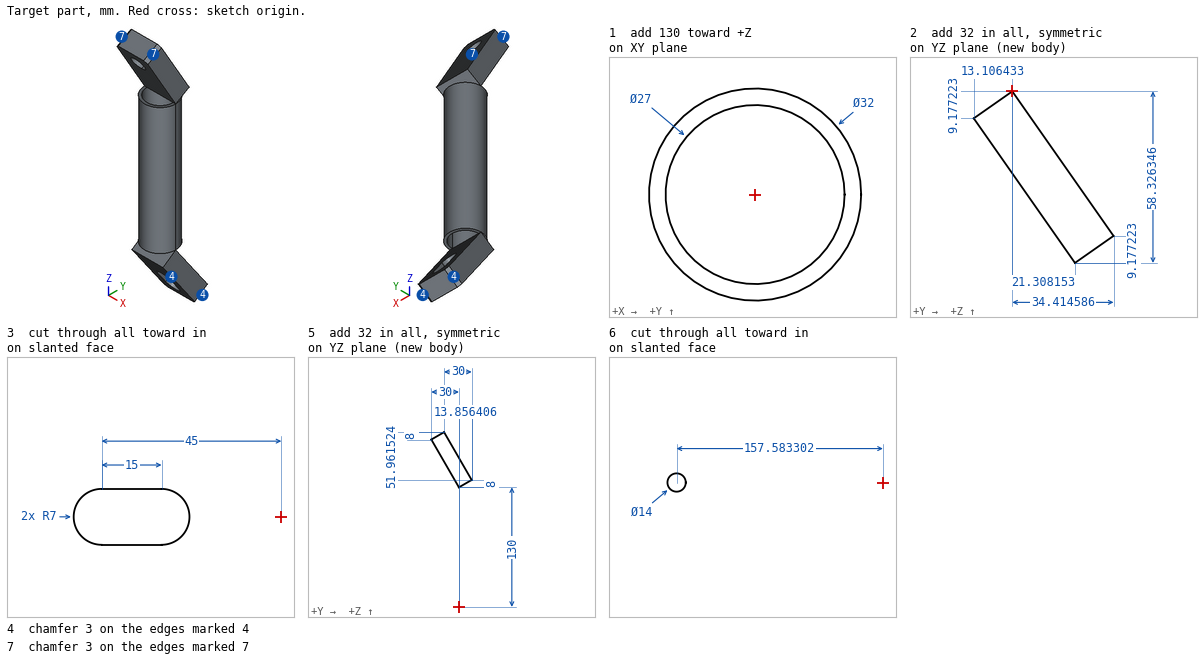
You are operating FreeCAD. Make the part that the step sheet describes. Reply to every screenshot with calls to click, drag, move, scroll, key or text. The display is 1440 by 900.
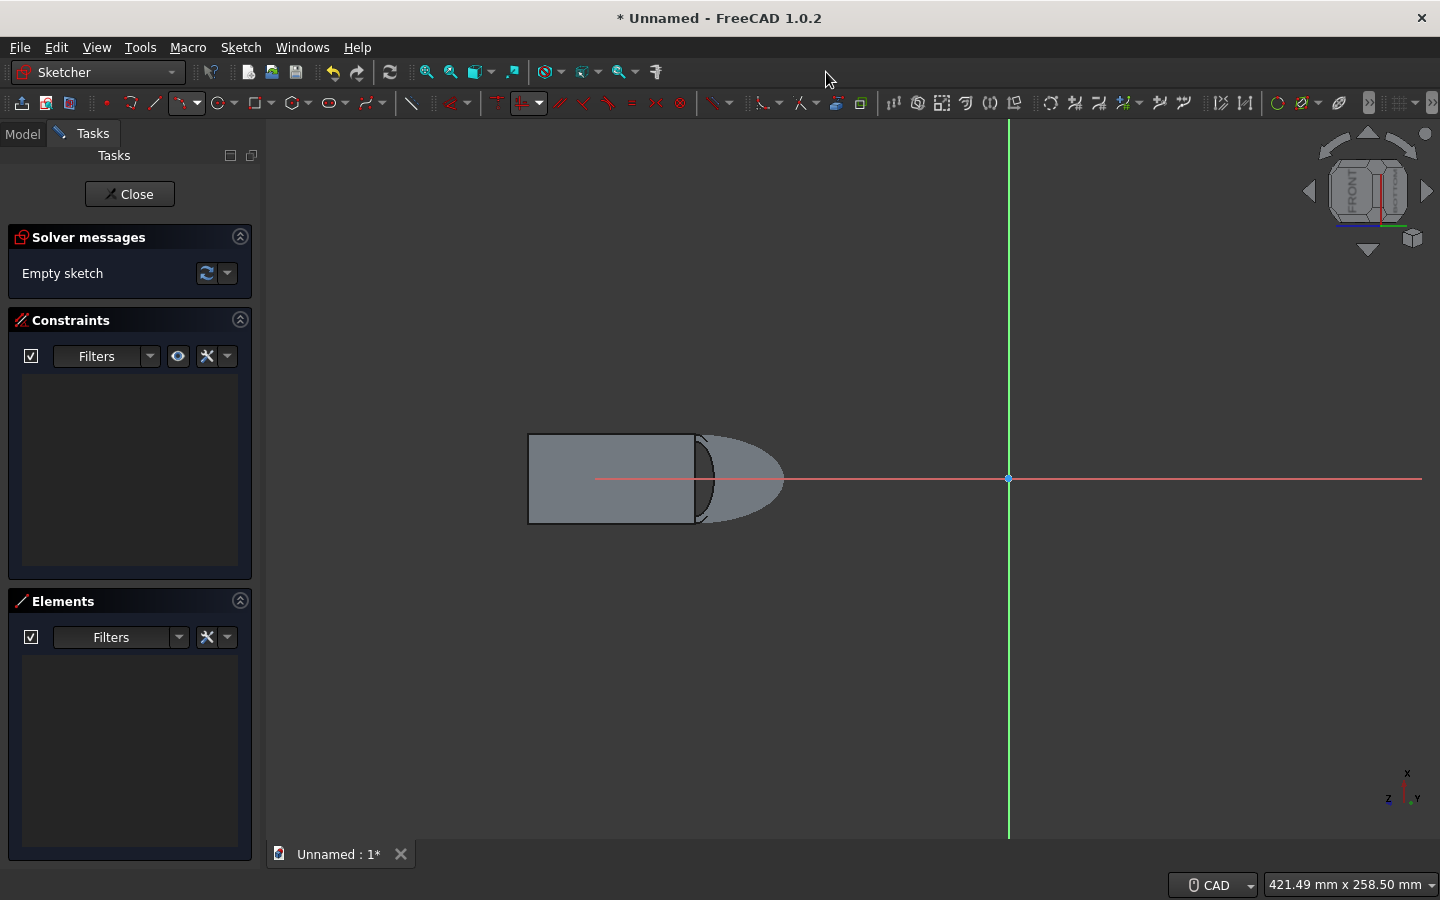
scroll(548, 479, up, 12)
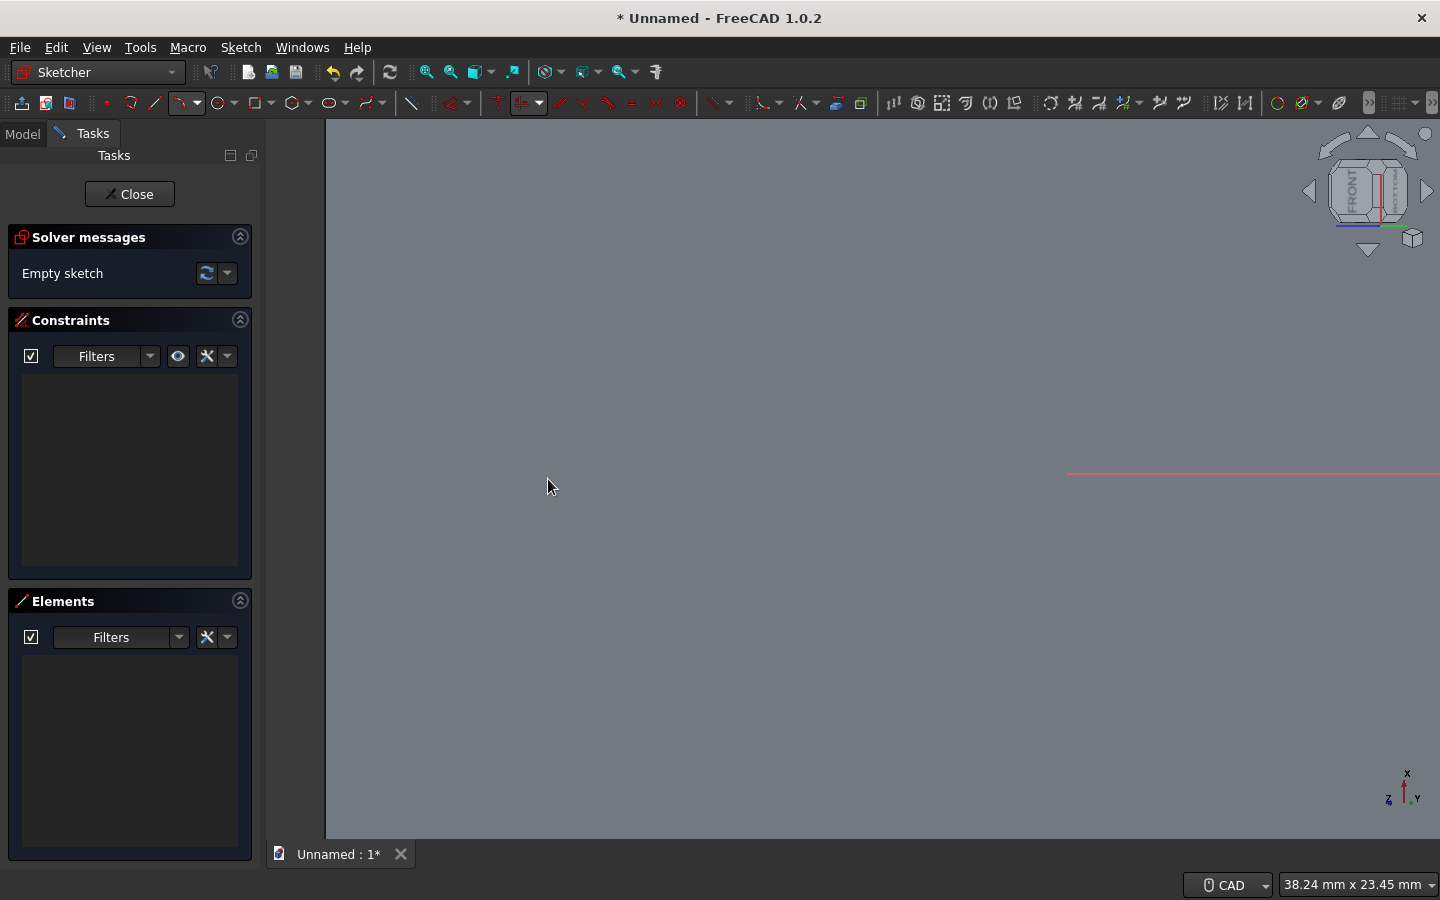
click(218, 104)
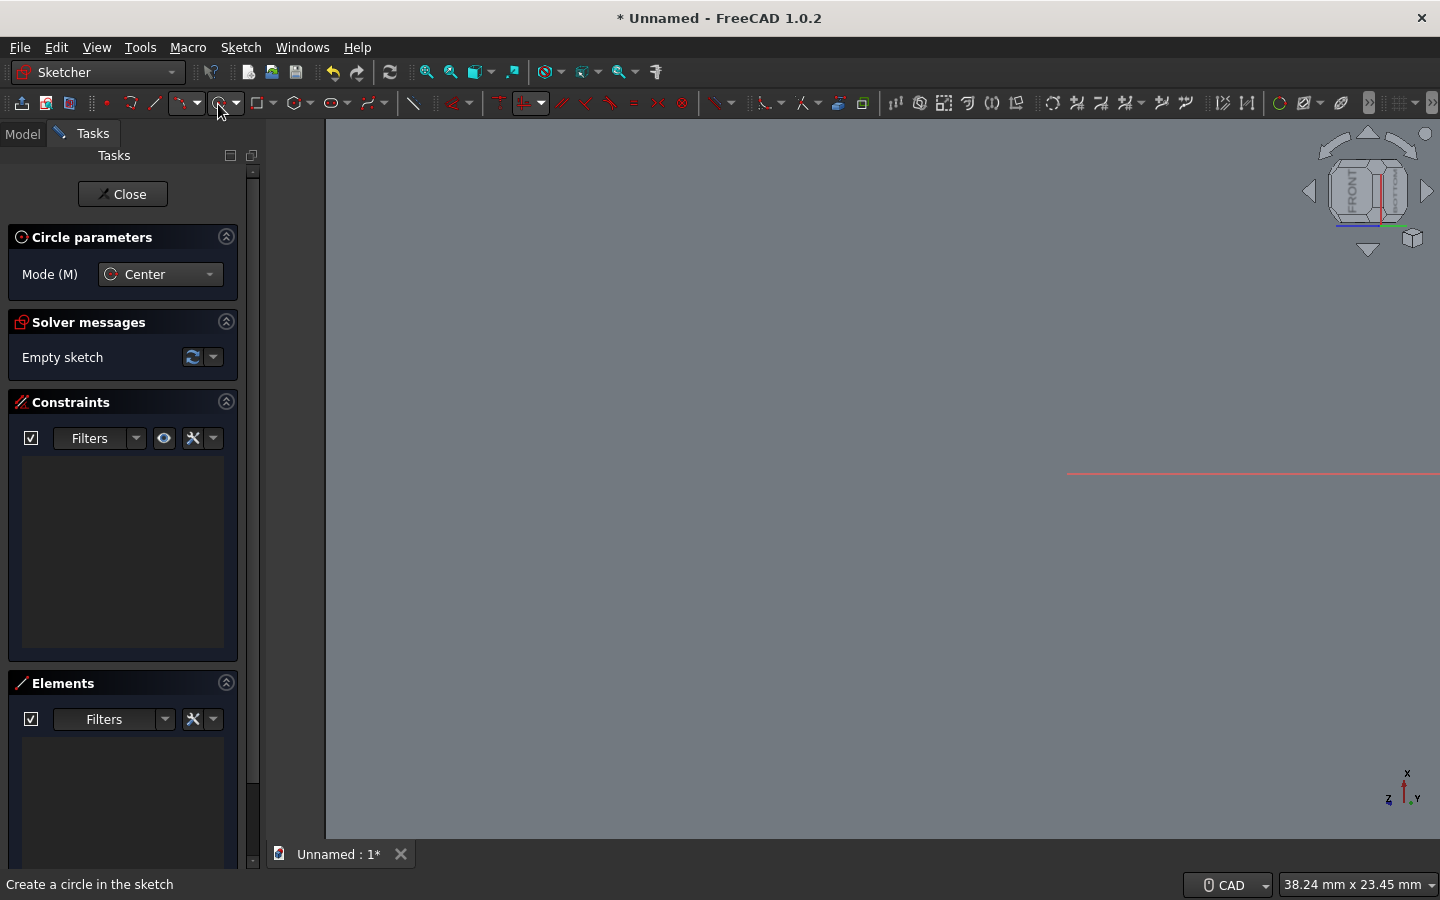
click(786, 474)
click(937, 322)
key(Escape)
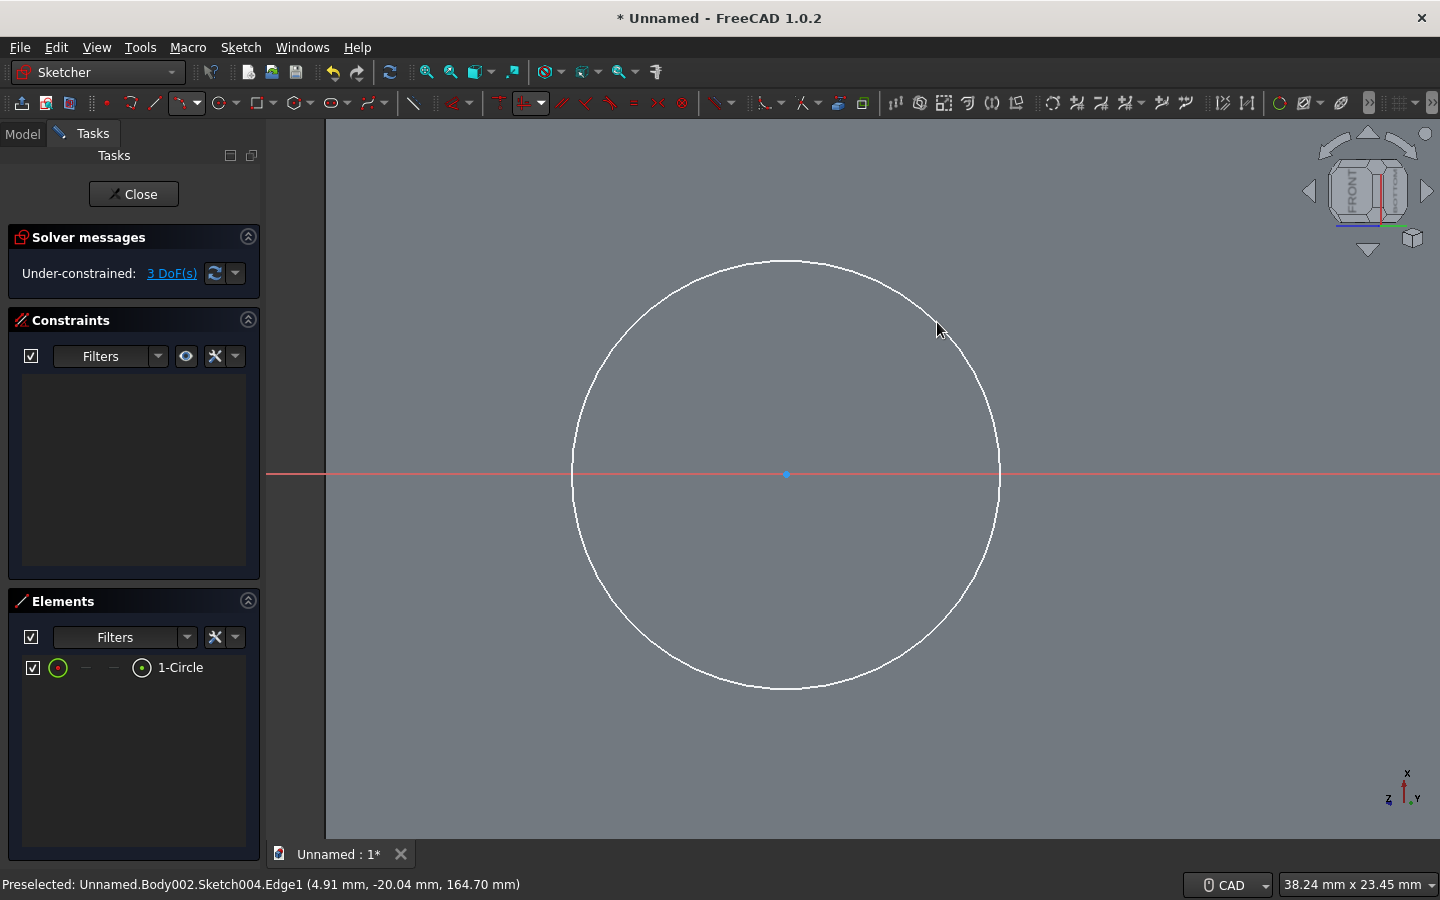
click(786, 475)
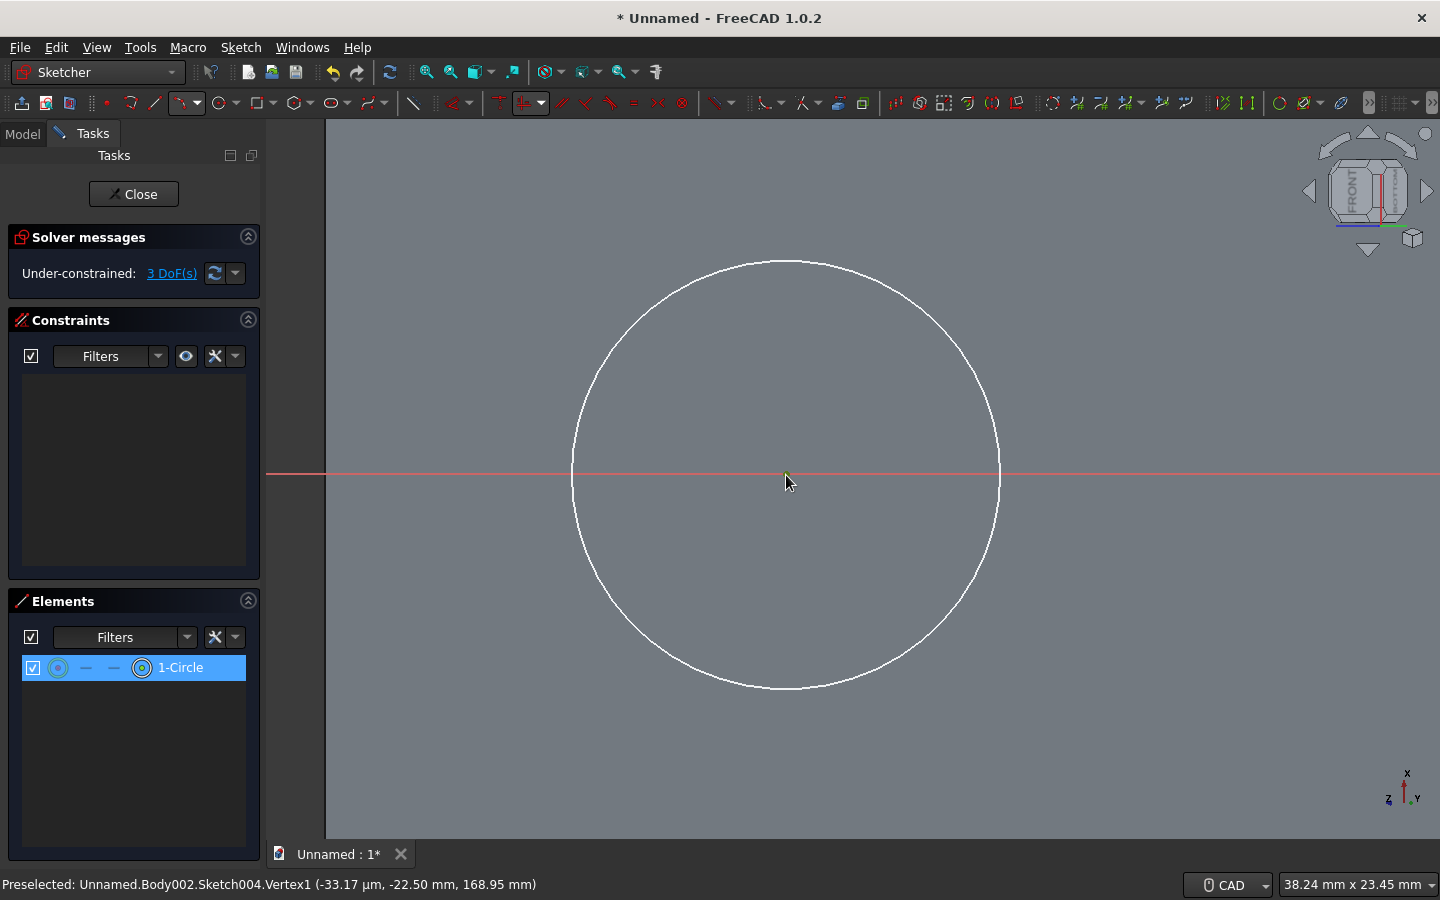
click(364, 474)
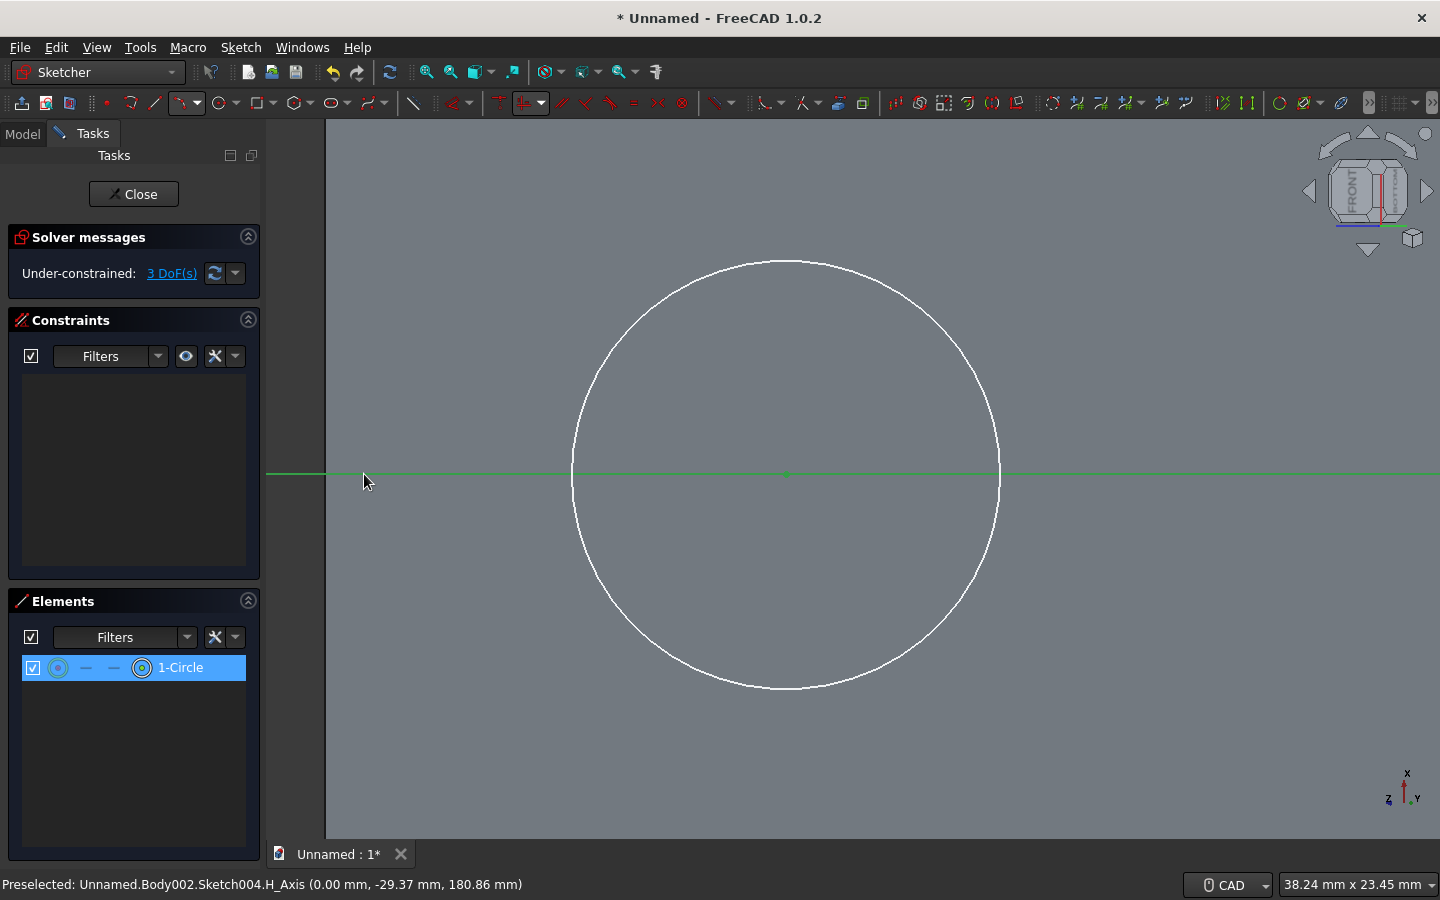
click(500, 104)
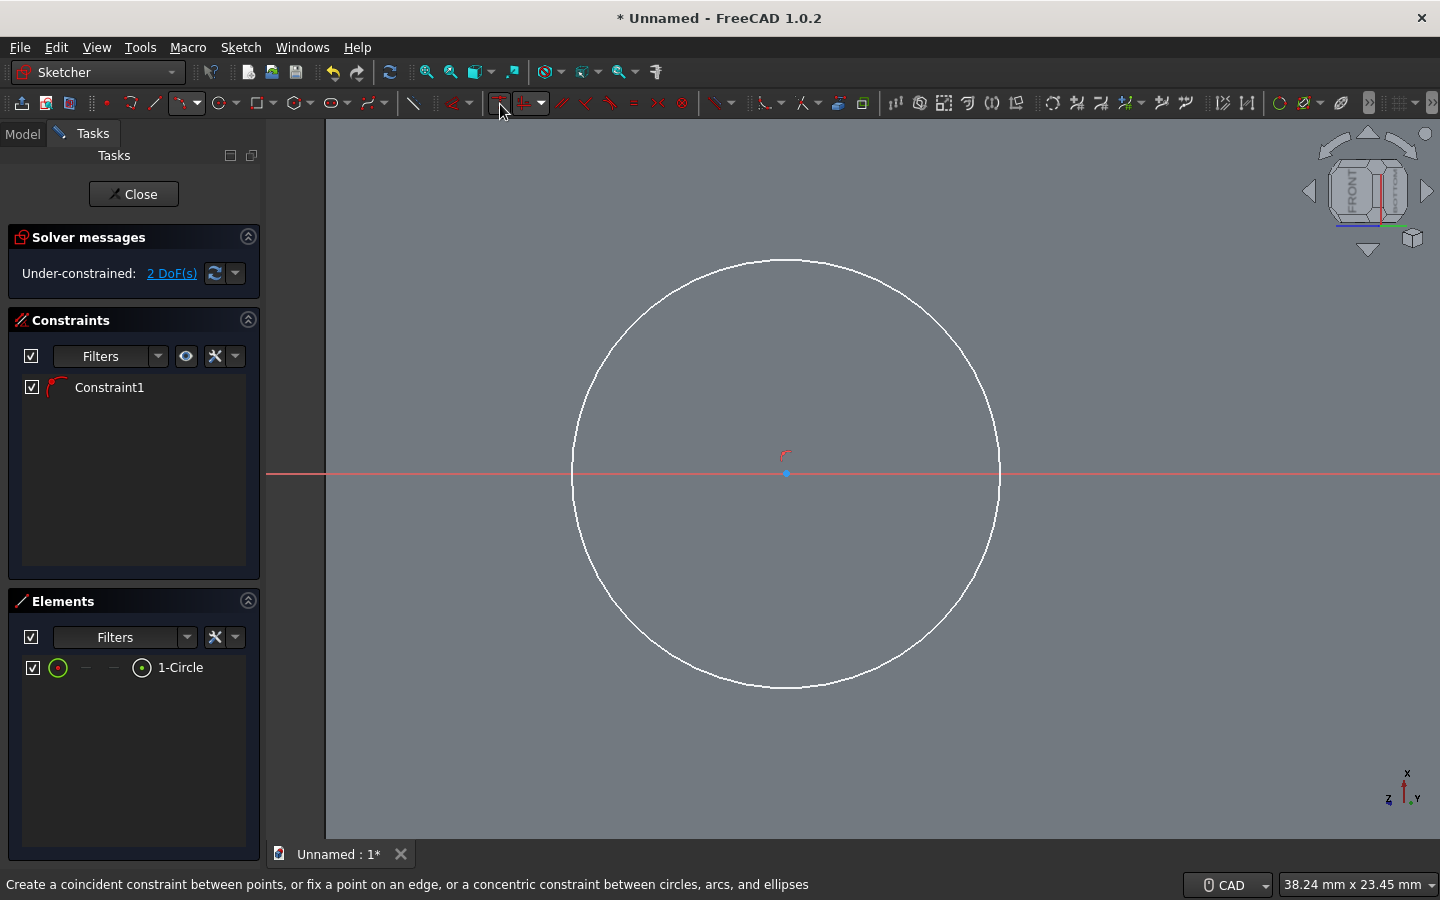
key(d)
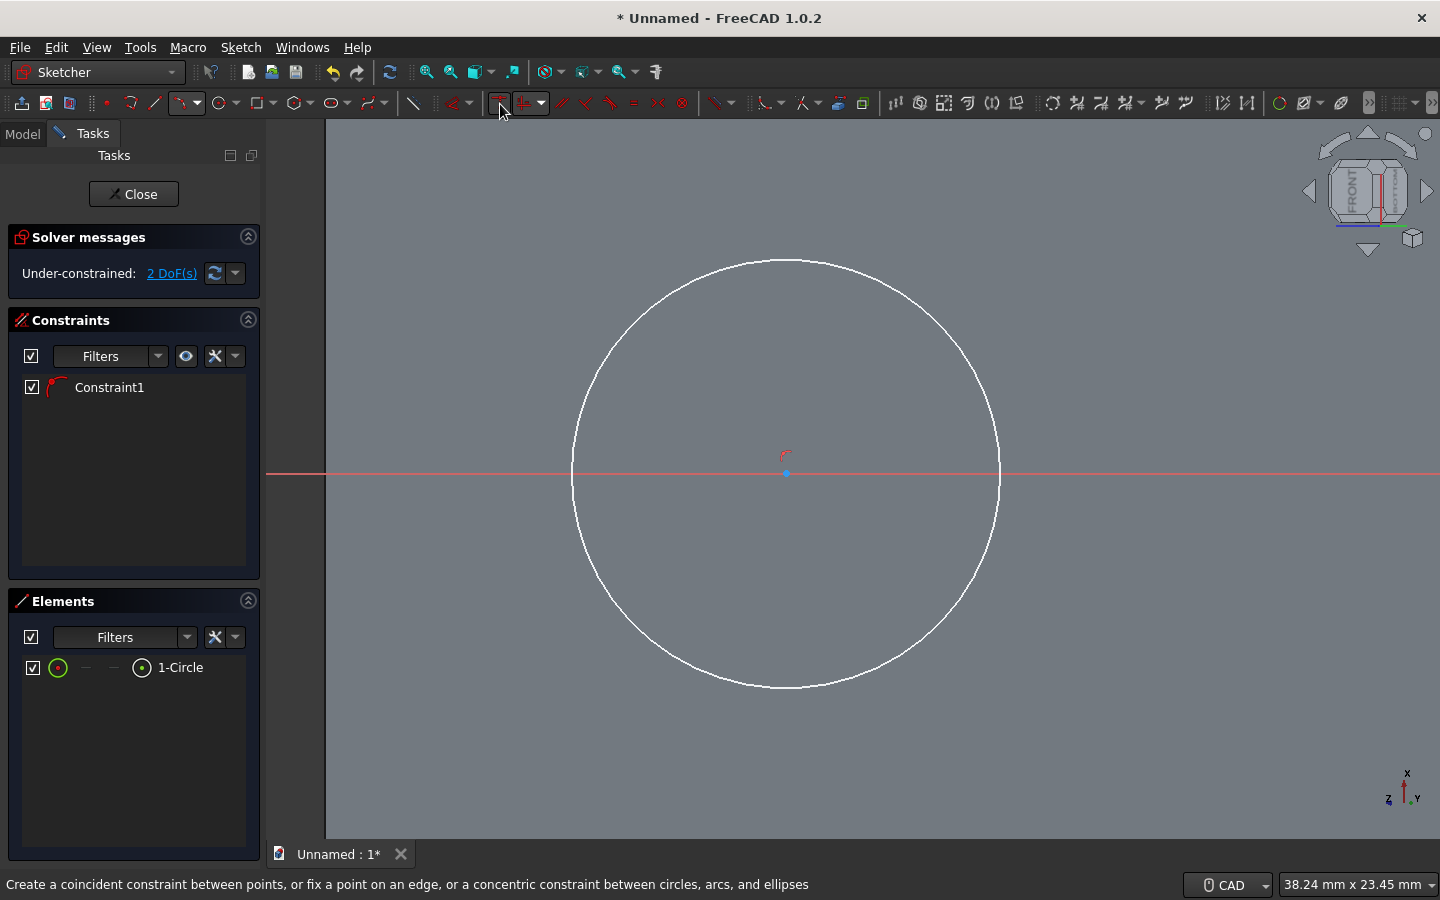
click(937, 322)
click(960, 299)